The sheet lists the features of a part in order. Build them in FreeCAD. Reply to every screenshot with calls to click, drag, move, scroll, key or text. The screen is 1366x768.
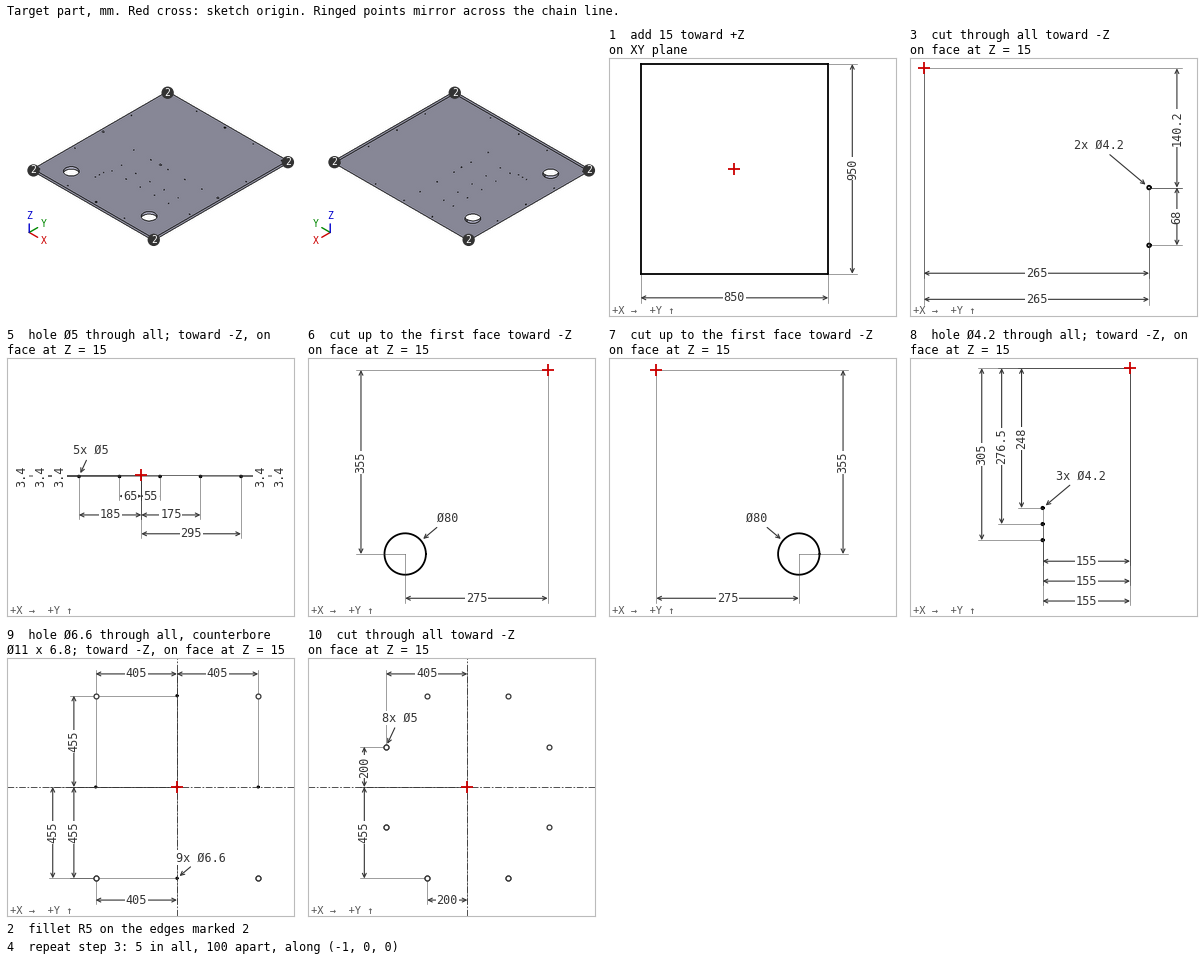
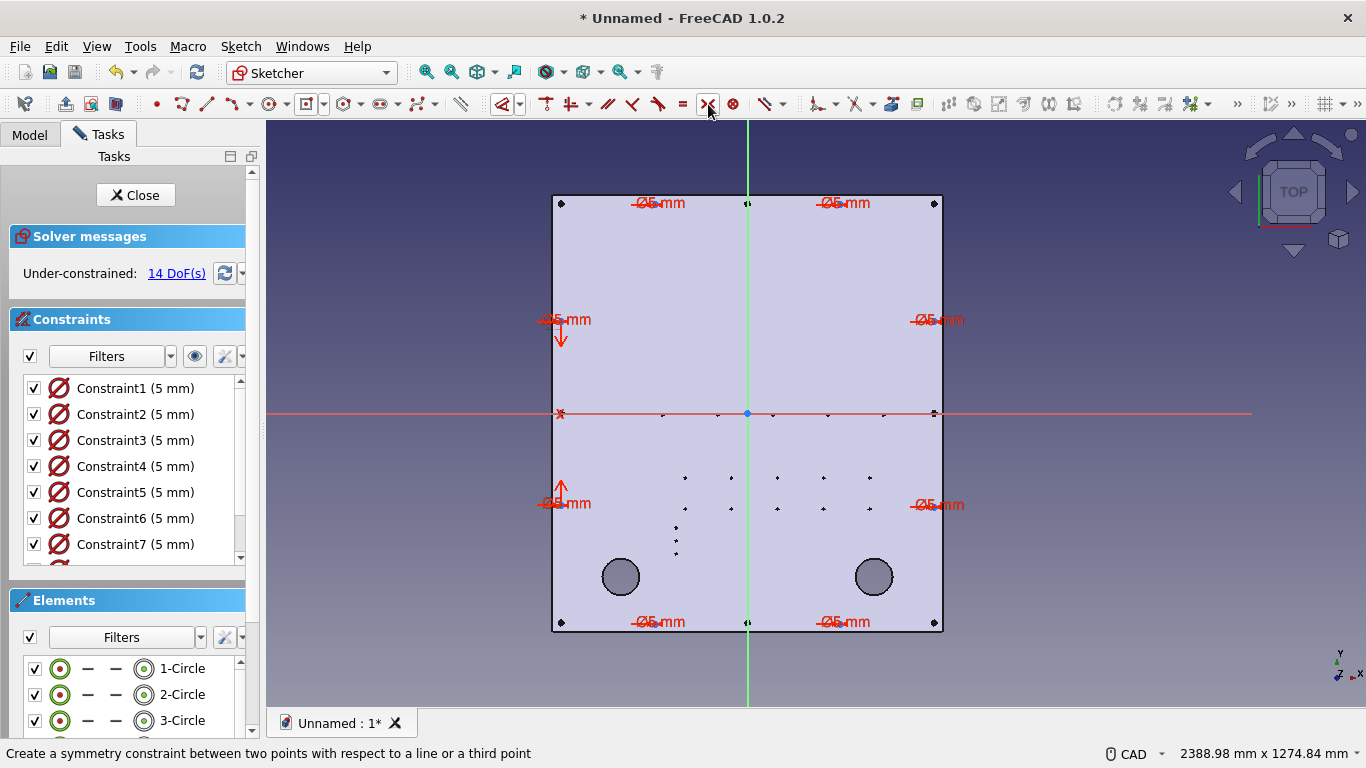
click(655, 624)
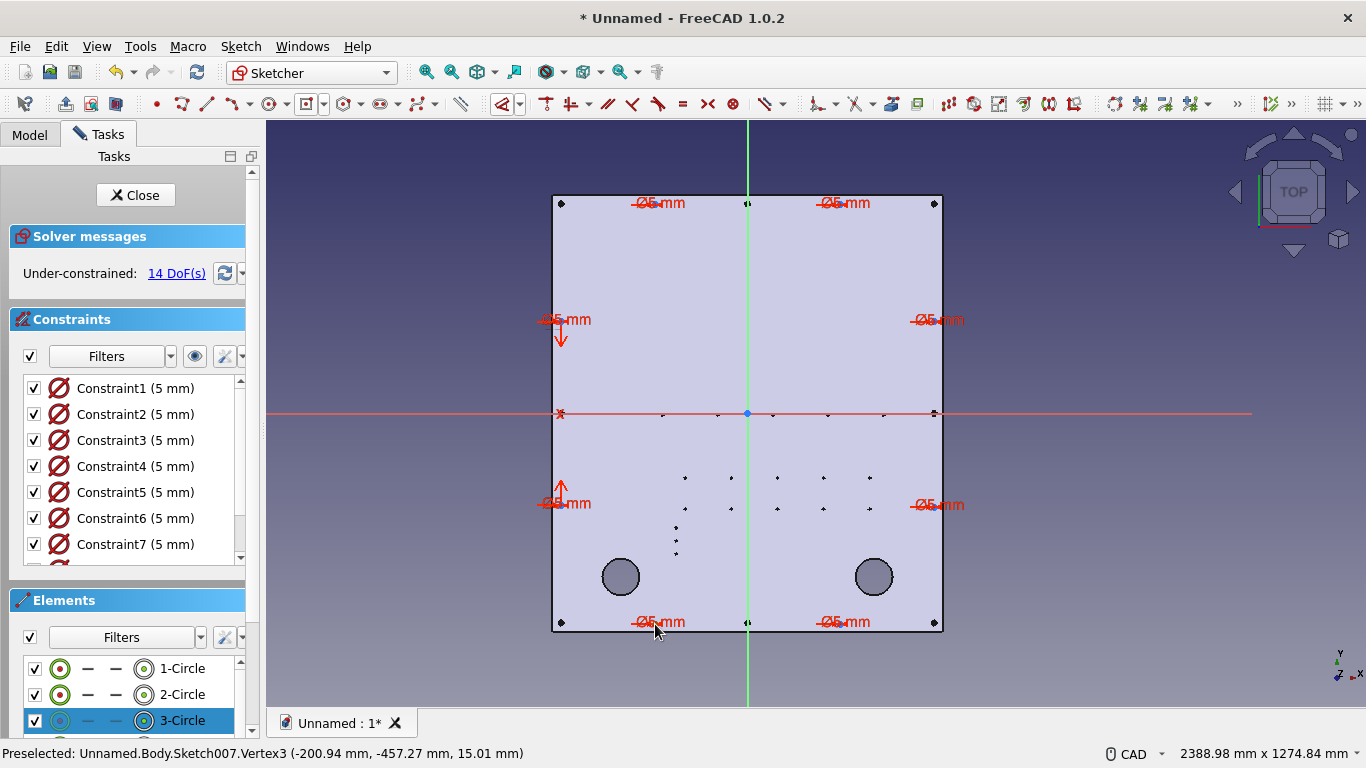
click(840, 624)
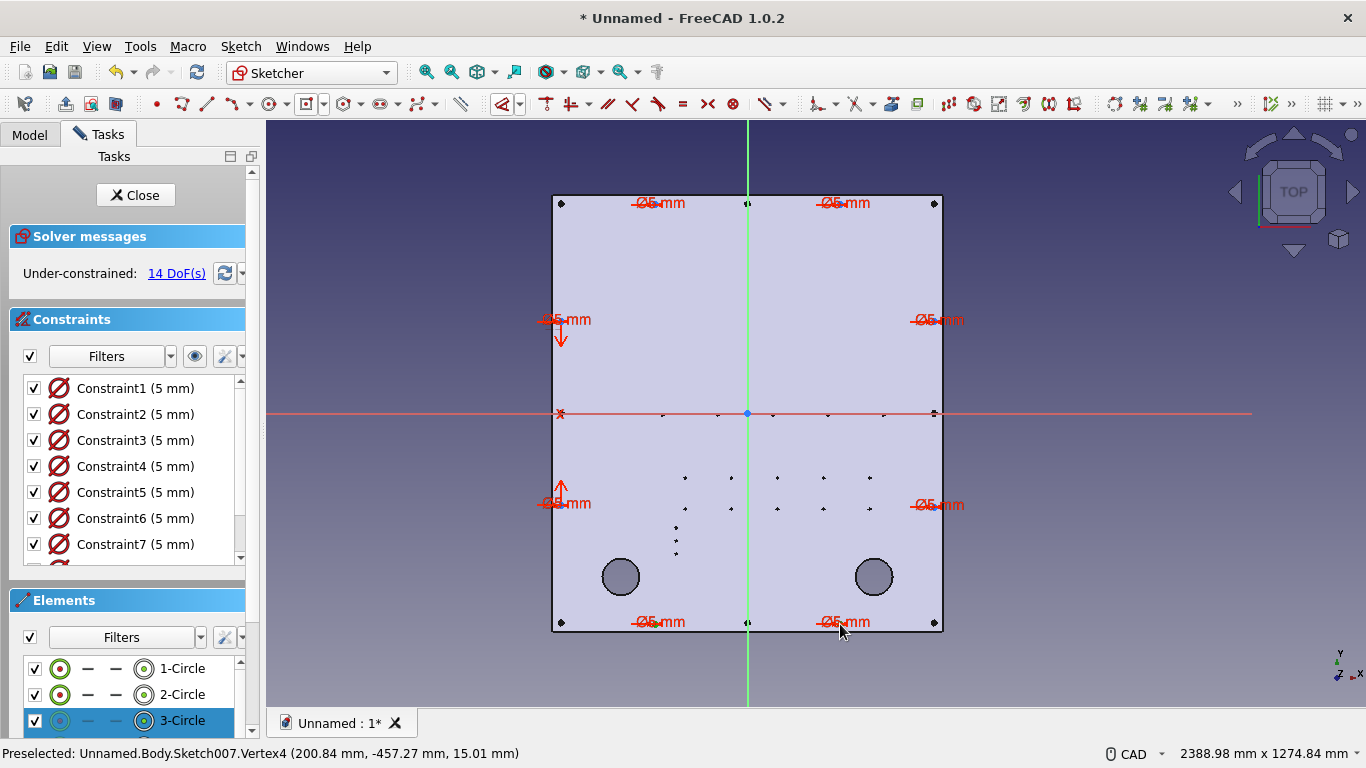
click(748, 641)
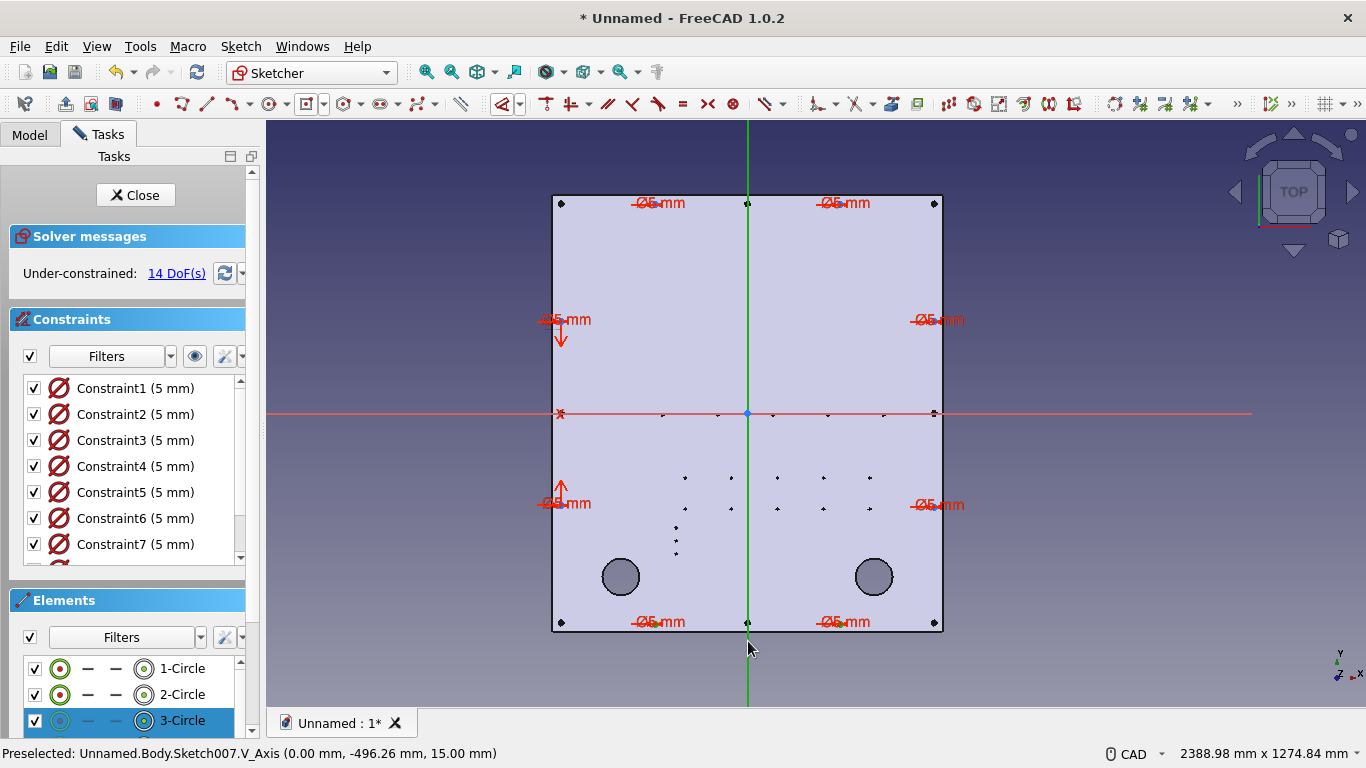
click(708, 104)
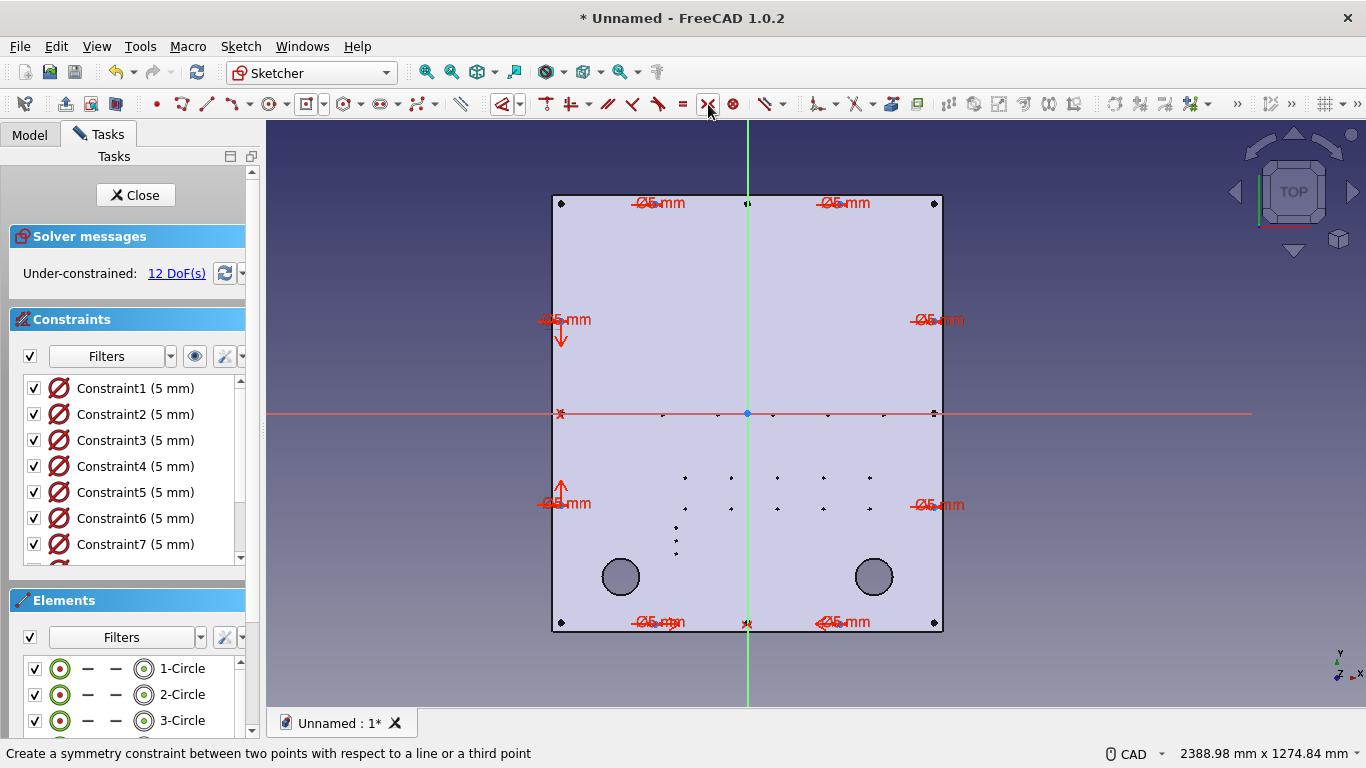
click(561, 505)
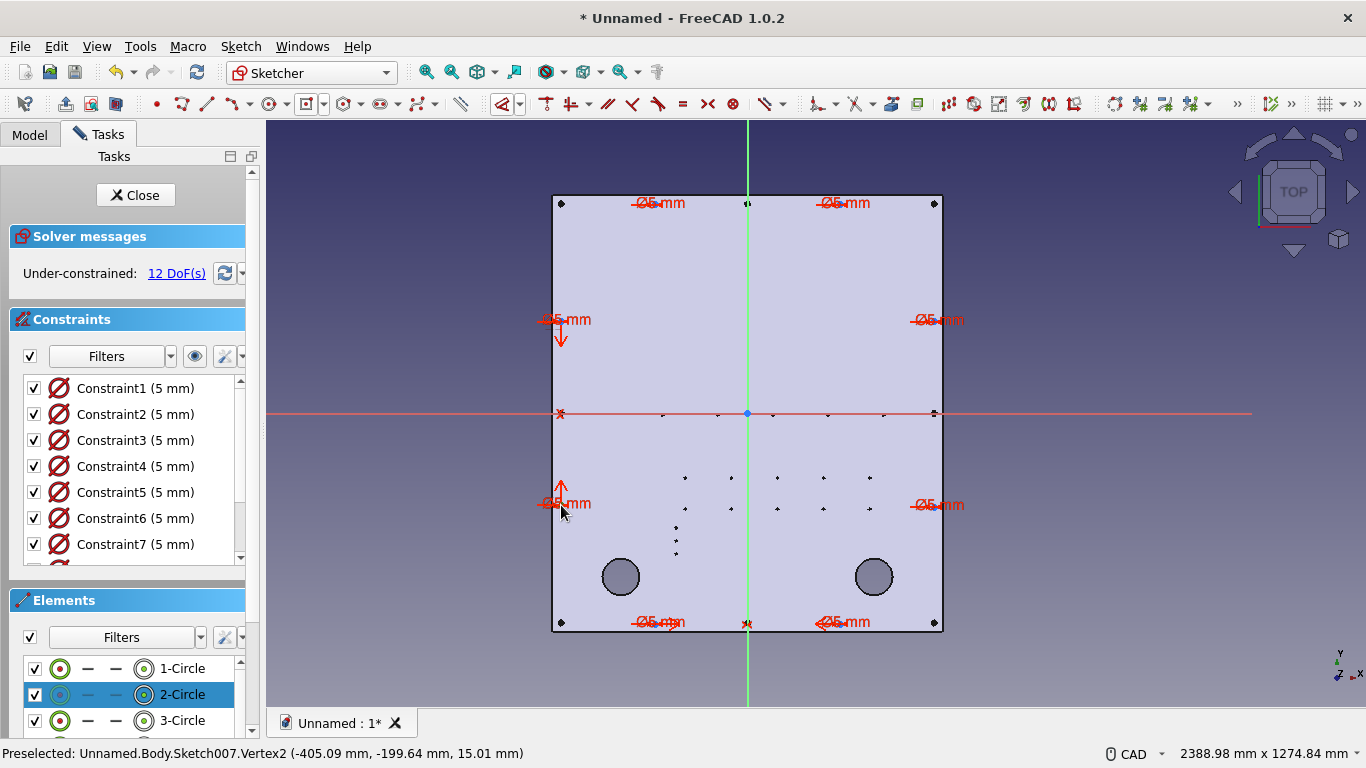
click(934, 507)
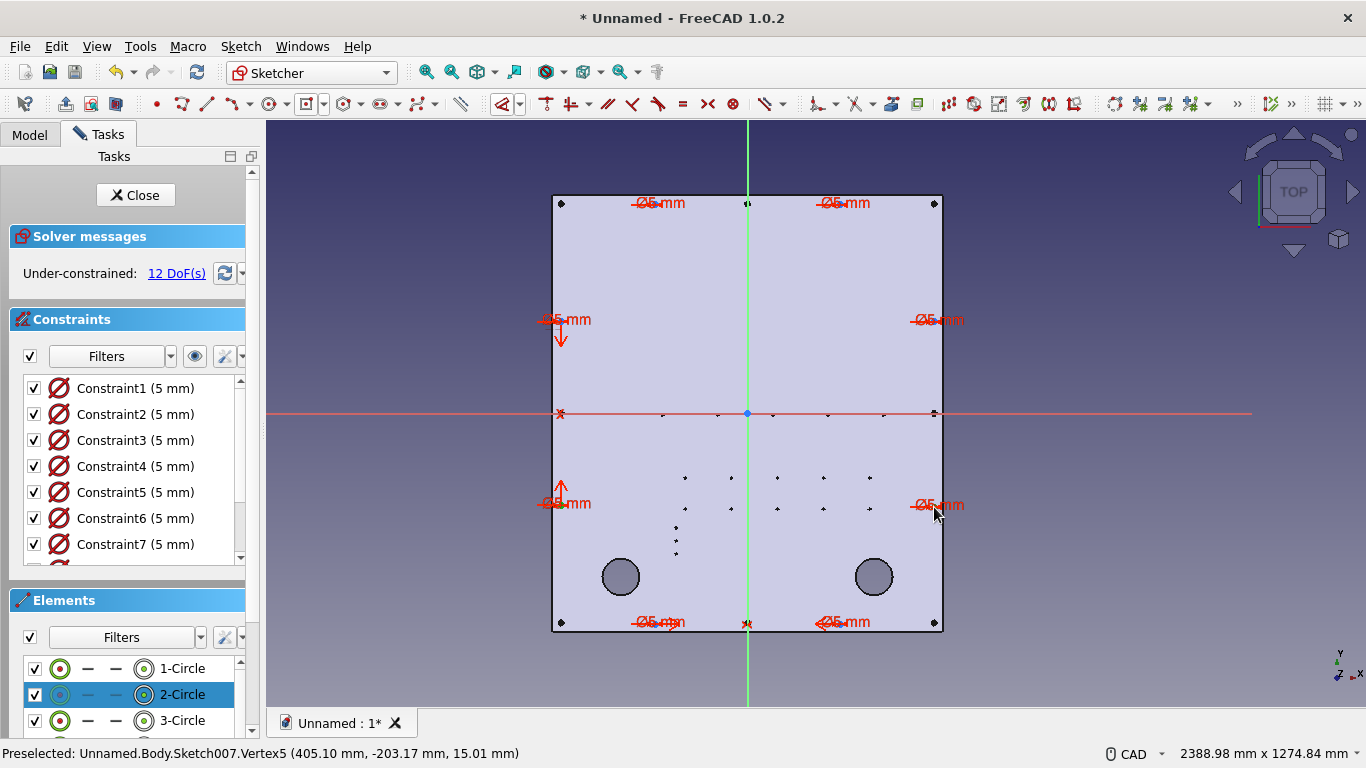
click(748, 641)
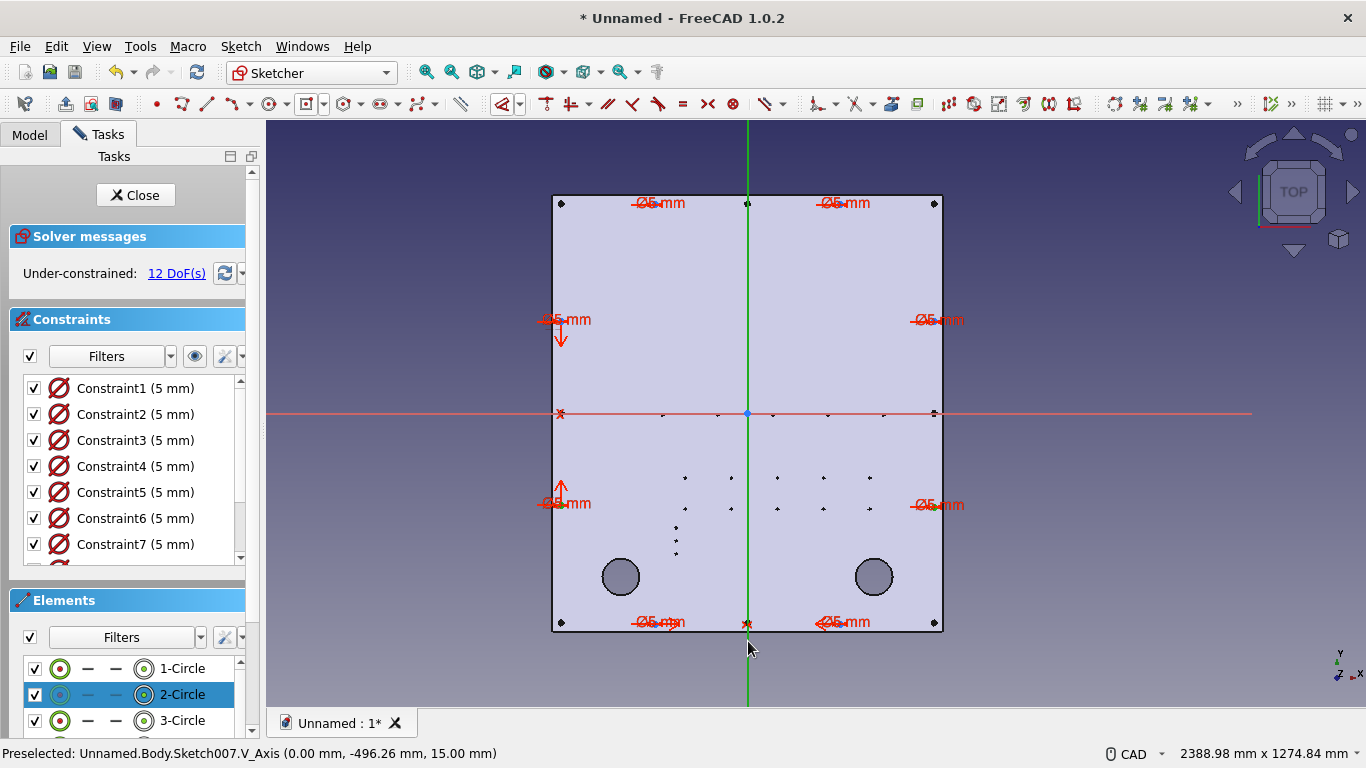
click(708, 104)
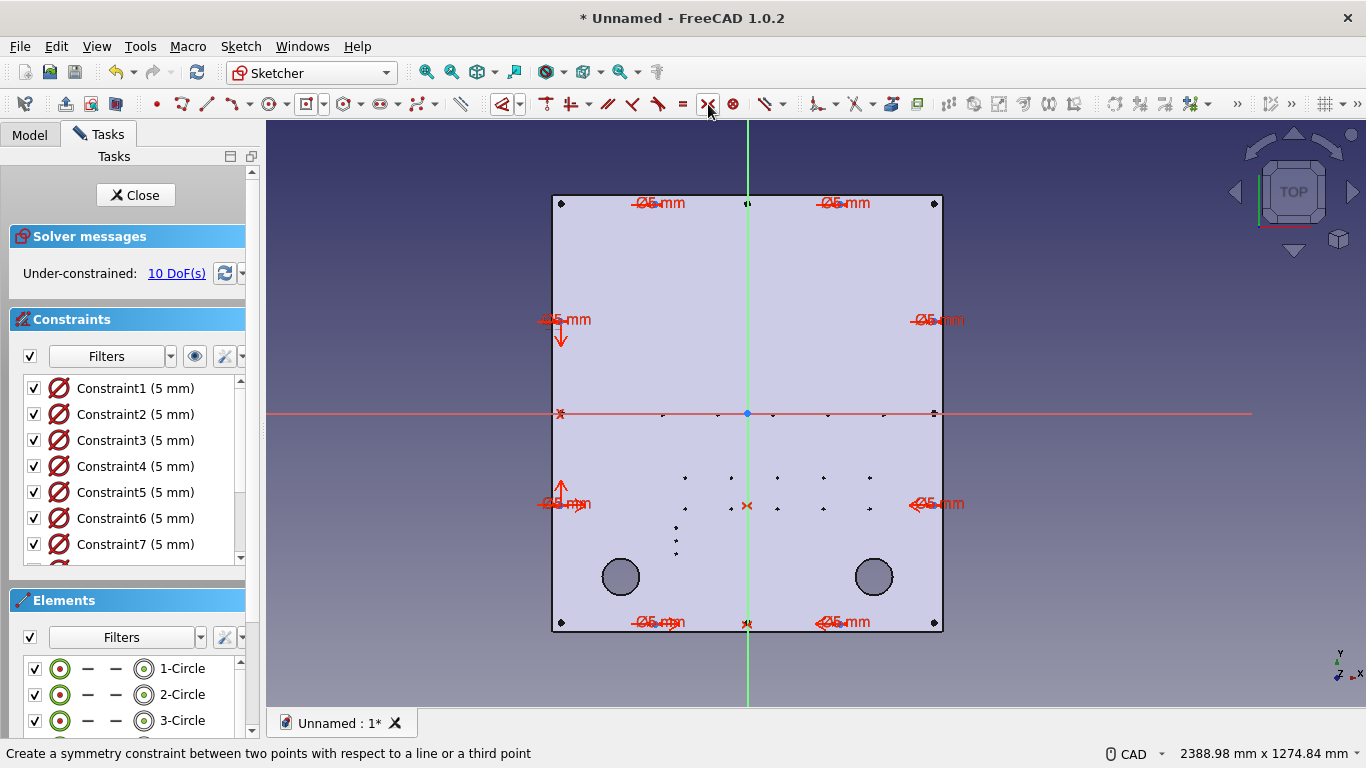
click(561, 322)